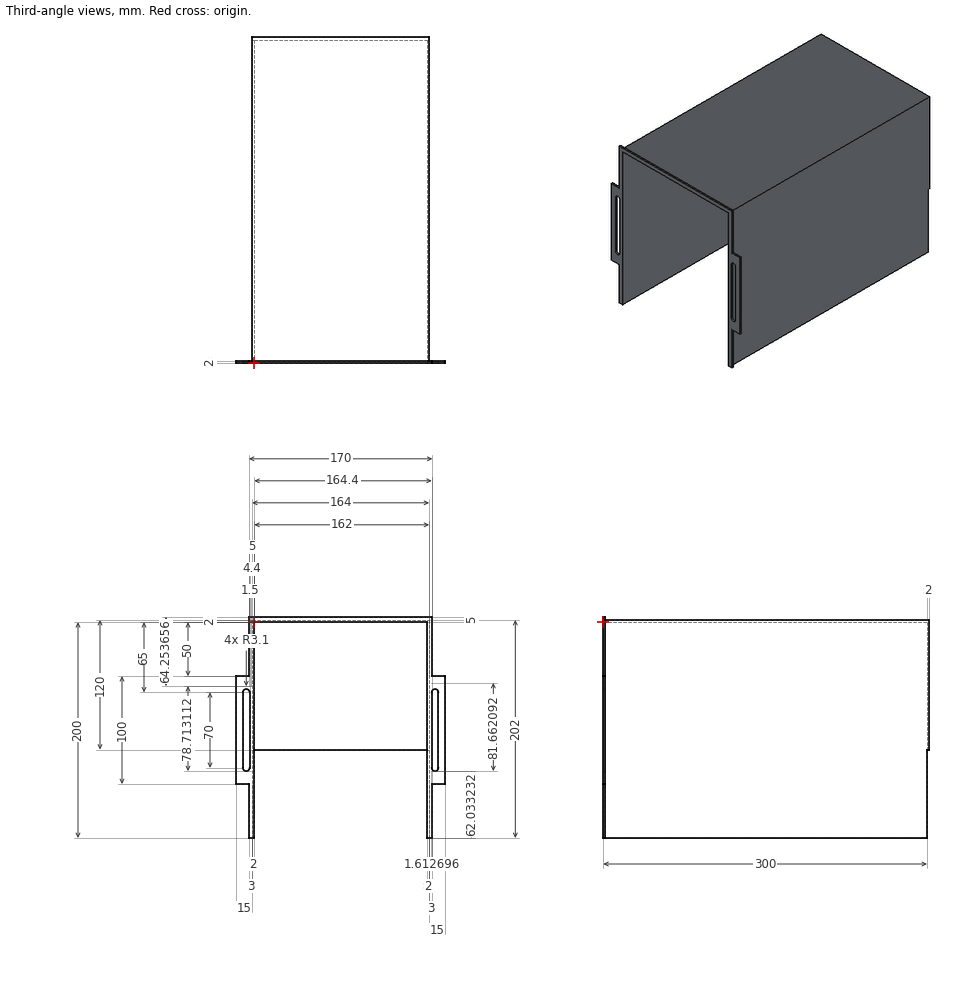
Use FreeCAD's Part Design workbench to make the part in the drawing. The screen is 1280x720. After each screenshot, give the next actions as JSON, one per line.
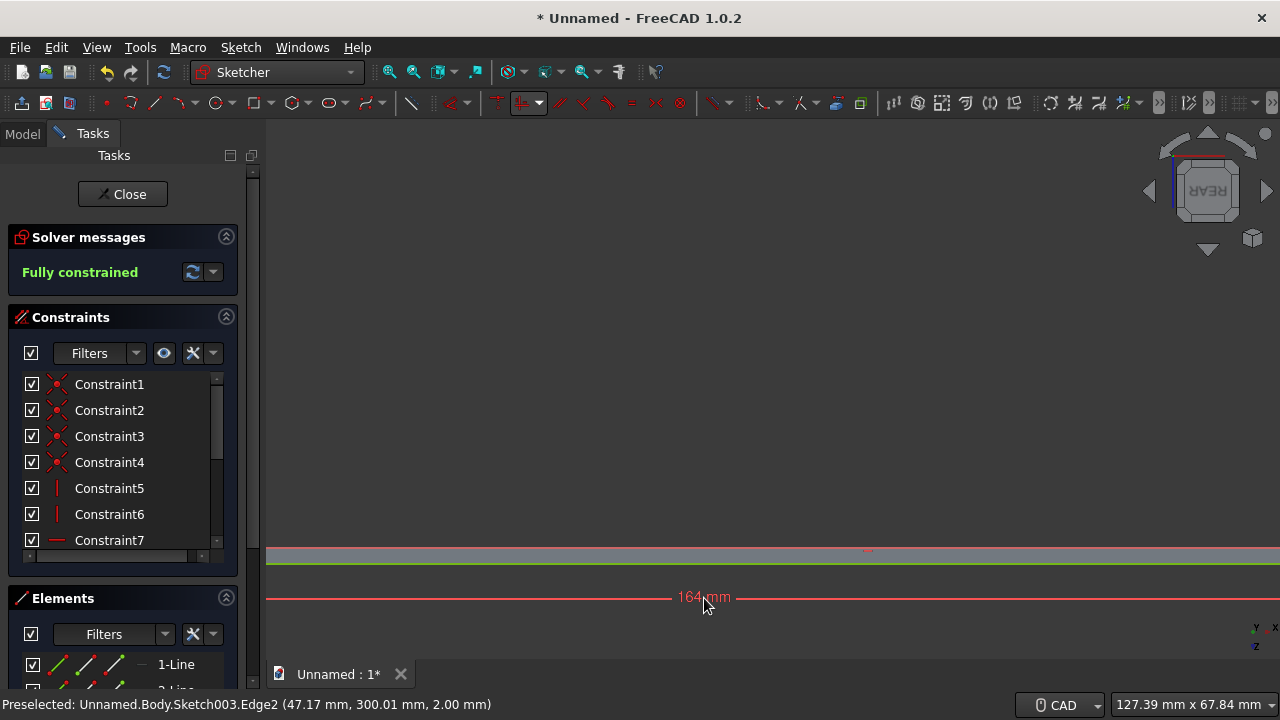
{"action": "left_click", "coordinate": [123, 194]}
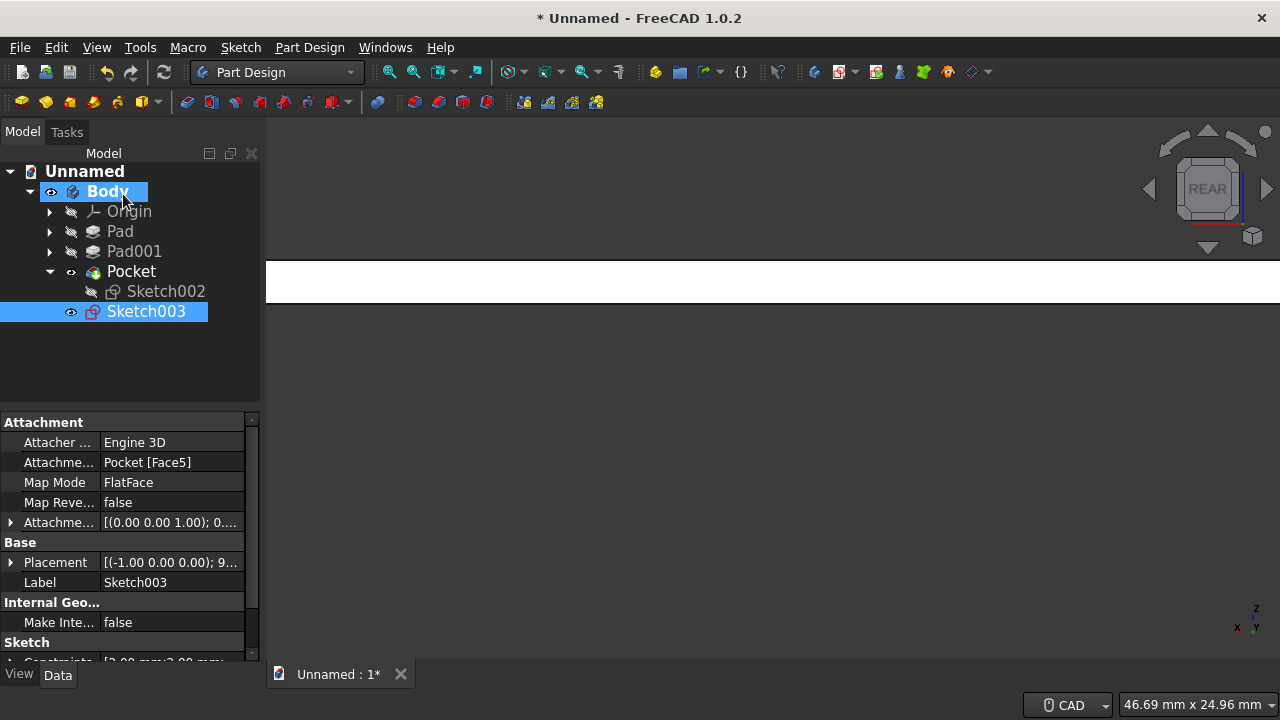
{"action": "left_click", "coordinate": [22, 102]}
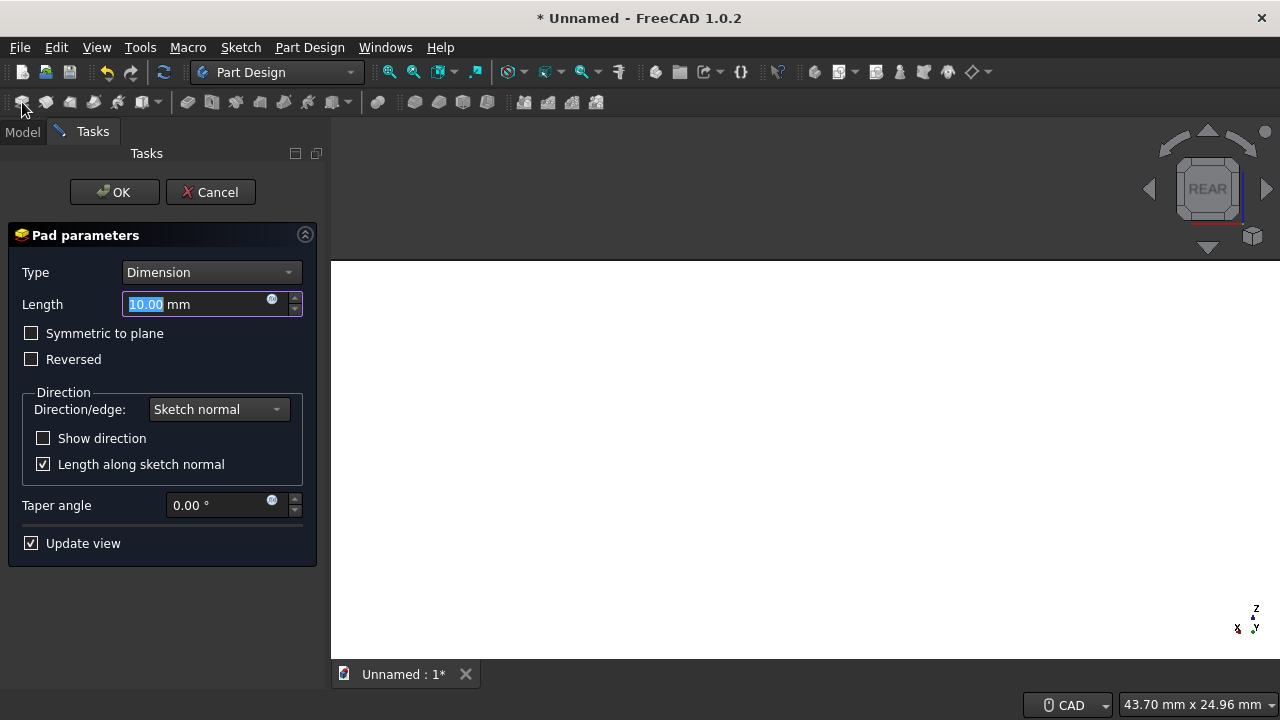
{"action": "type", "text": "2"}
{"action": "key", "text": "Tab"}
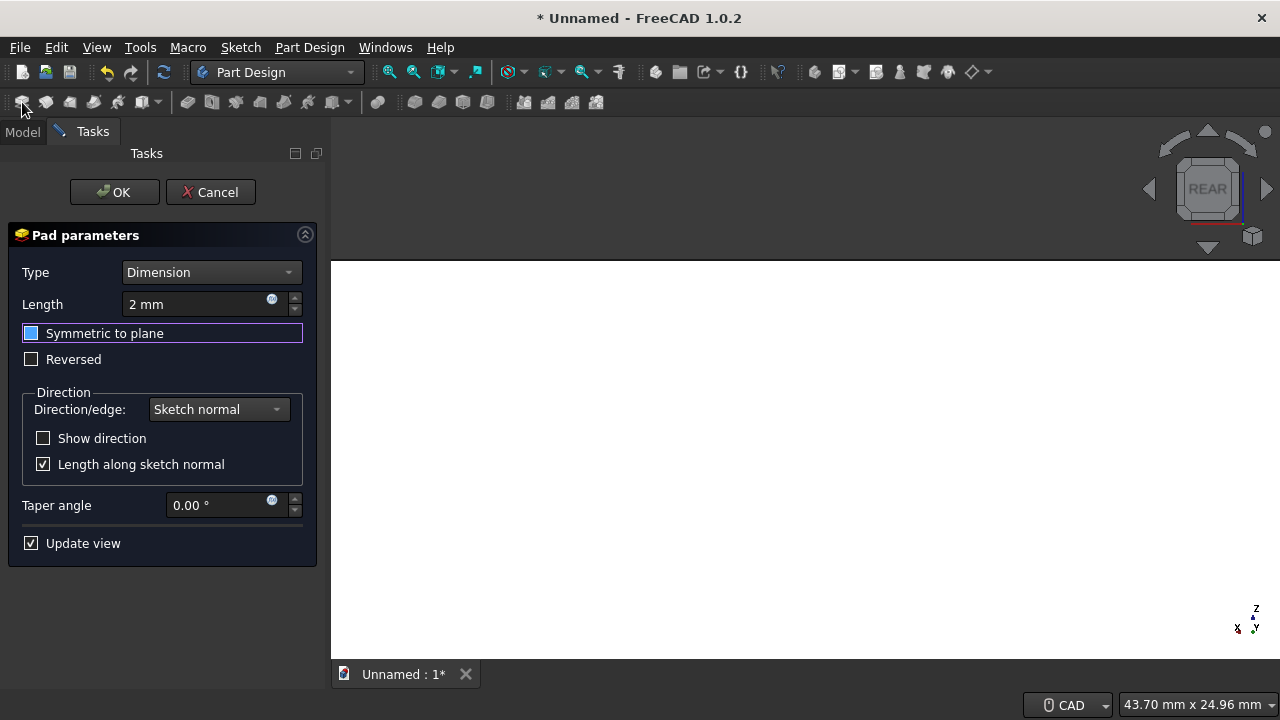
{"action": "left_click", "coordinate": [115, 192]}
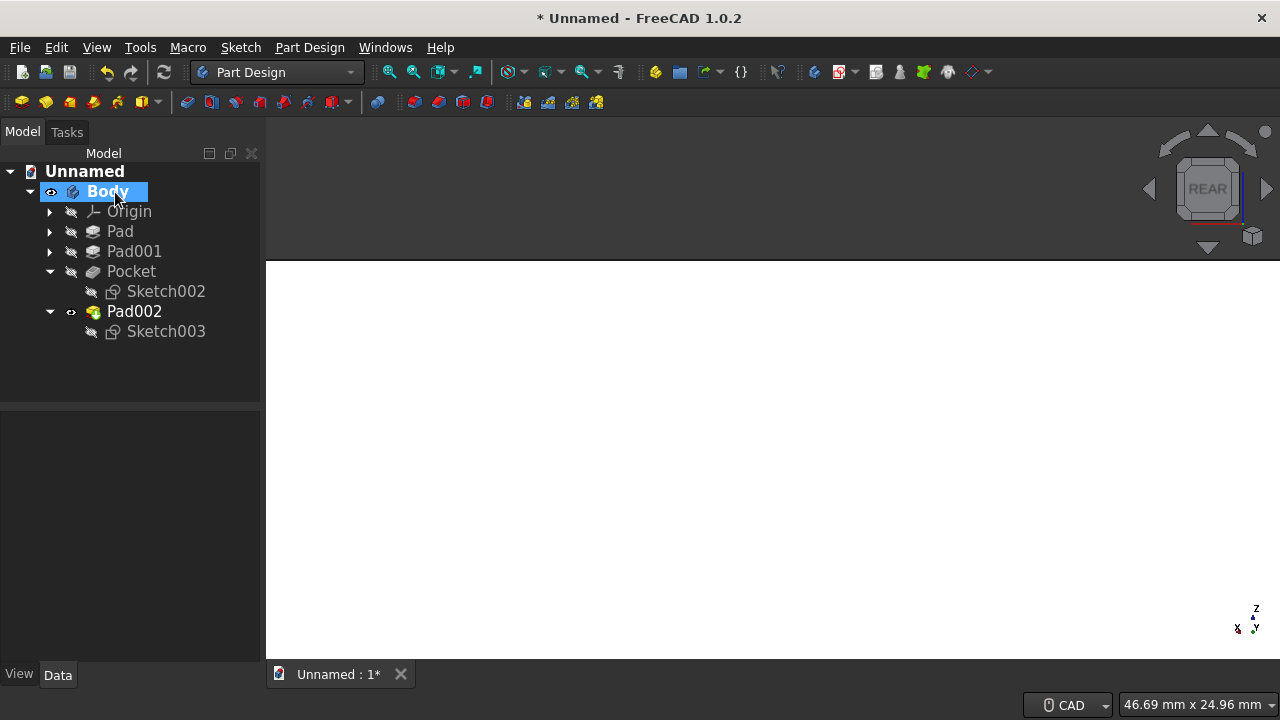
{"action": "left_click", "coordinate": [390, 72]}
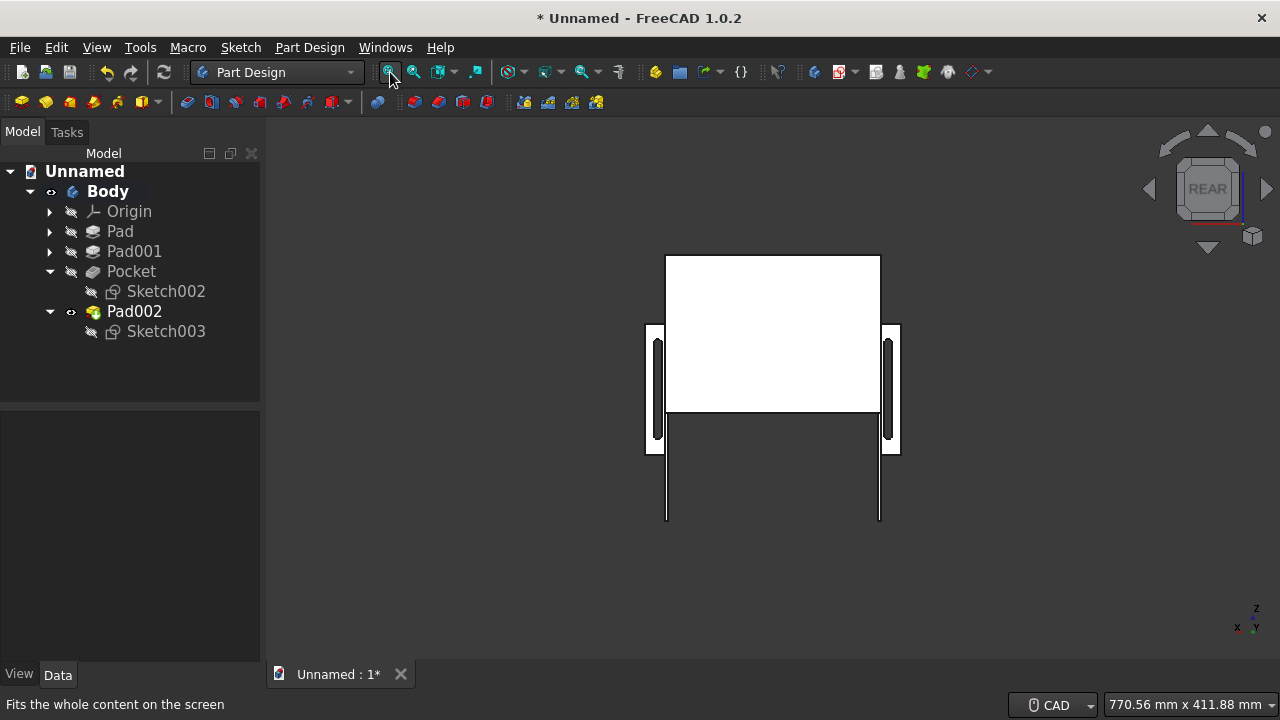
{"action": "key", "text": "0"}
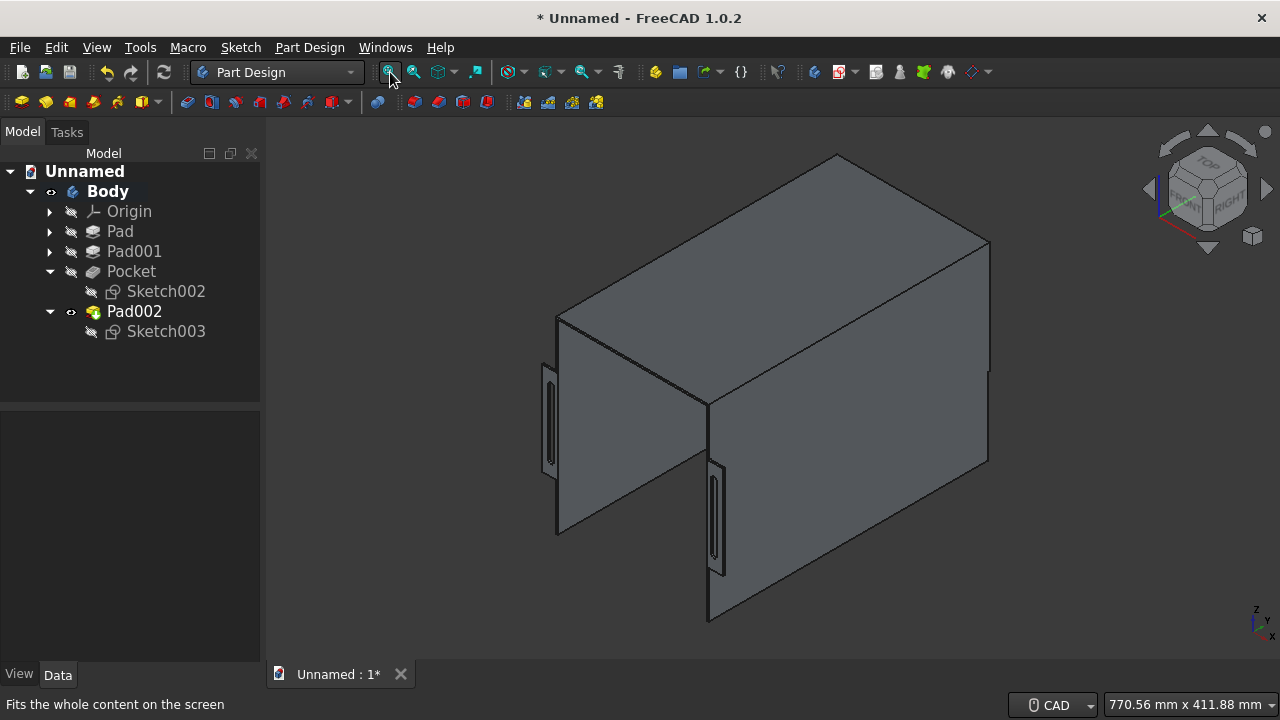
{"action": "scroll", "coordinate": [555, 454], "scroll_direction": "up", "scroll_amount": 10}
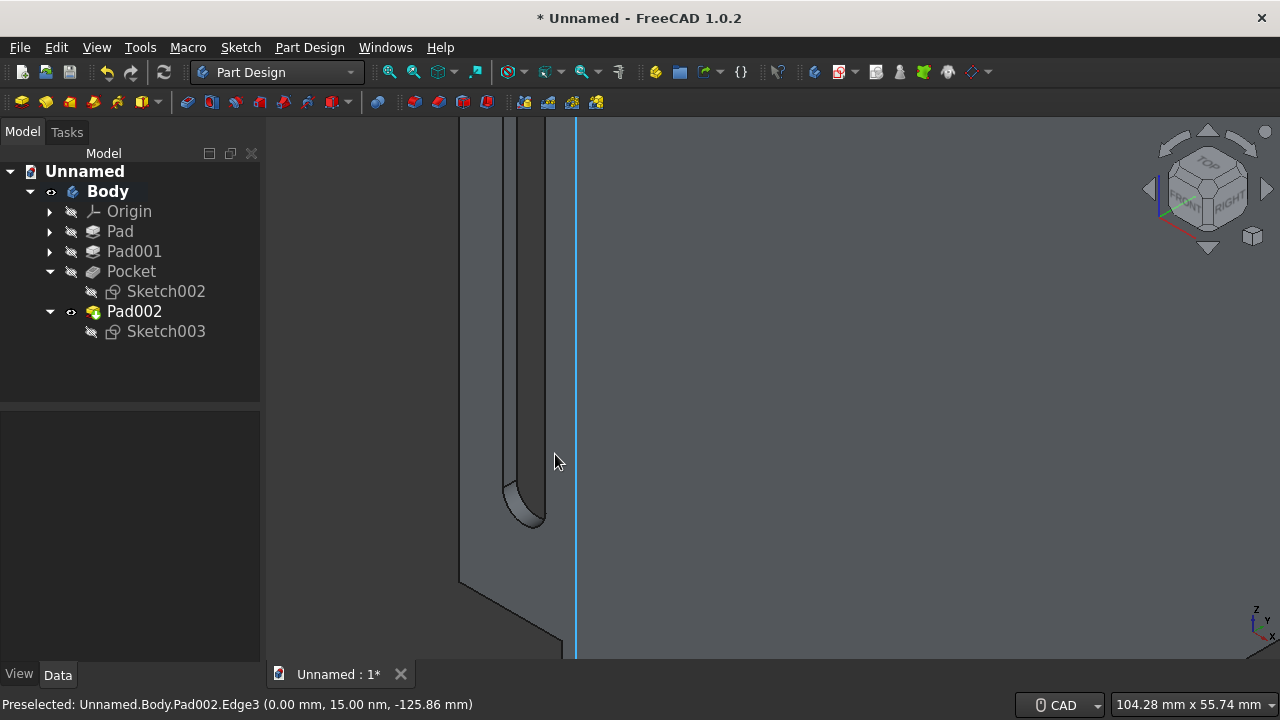
{"action": "left_click", "coordinate": [554, 460]}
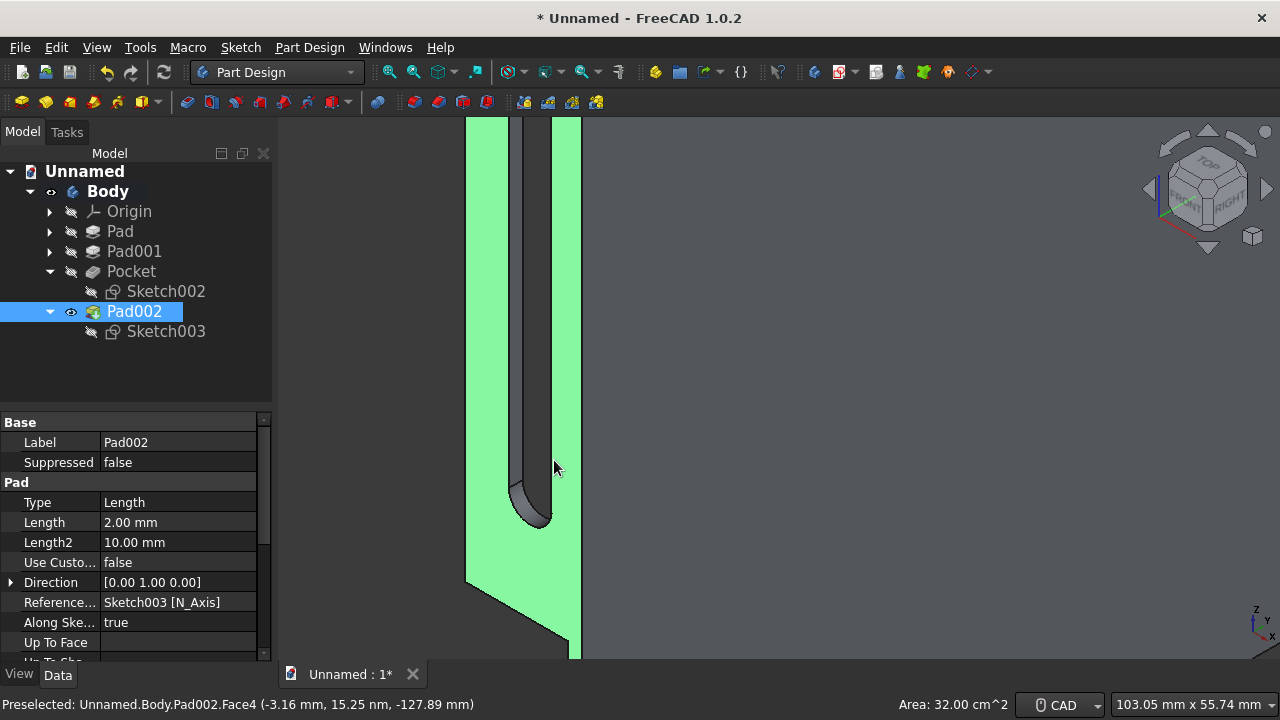
{"action": "left_click", "coordinate": [840, 72]}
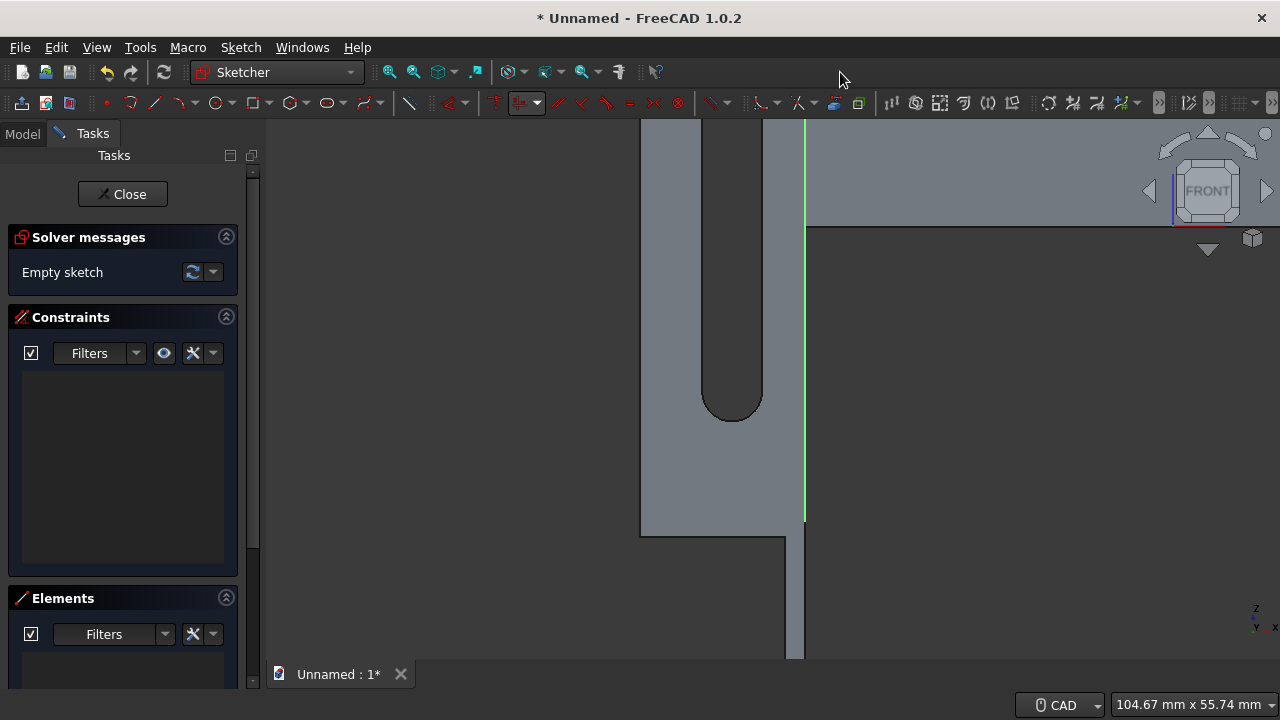
{"action": "scroll", "coordinate": [531, 460], "scroll_direction": "down", "scroll_amount": 9}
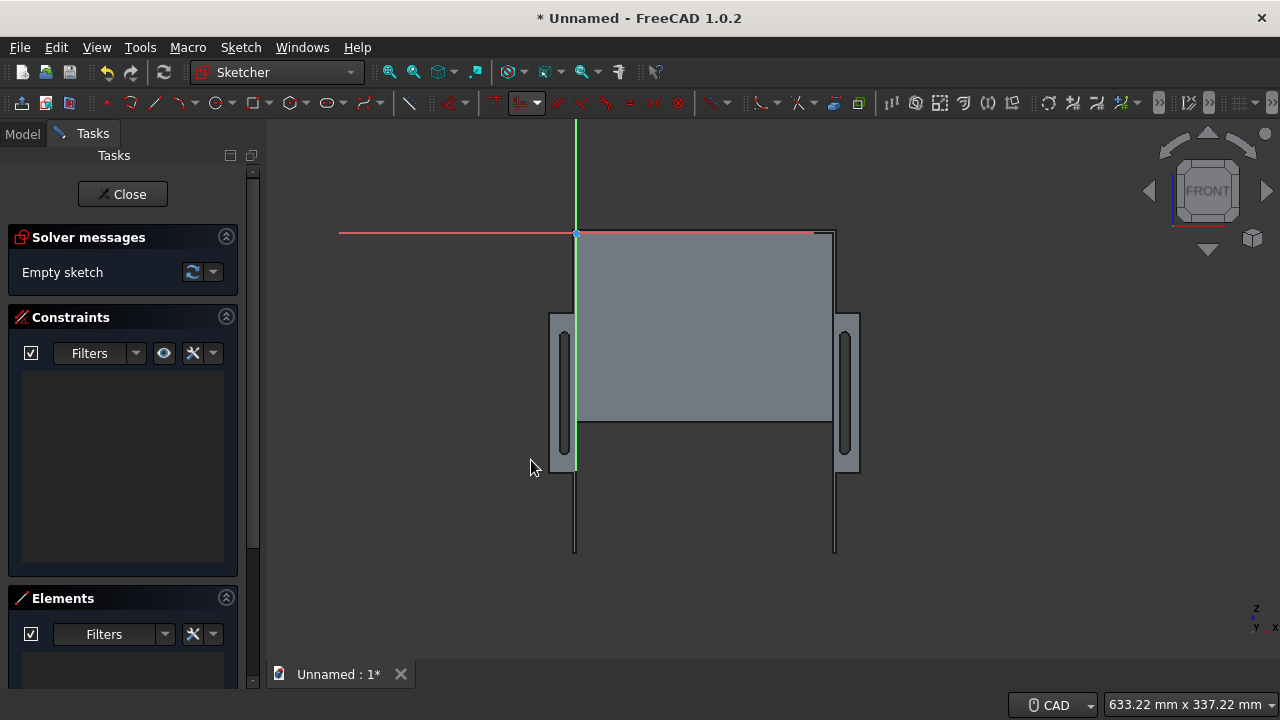
{"action": "left_click", "coordinate": [132, 104]}